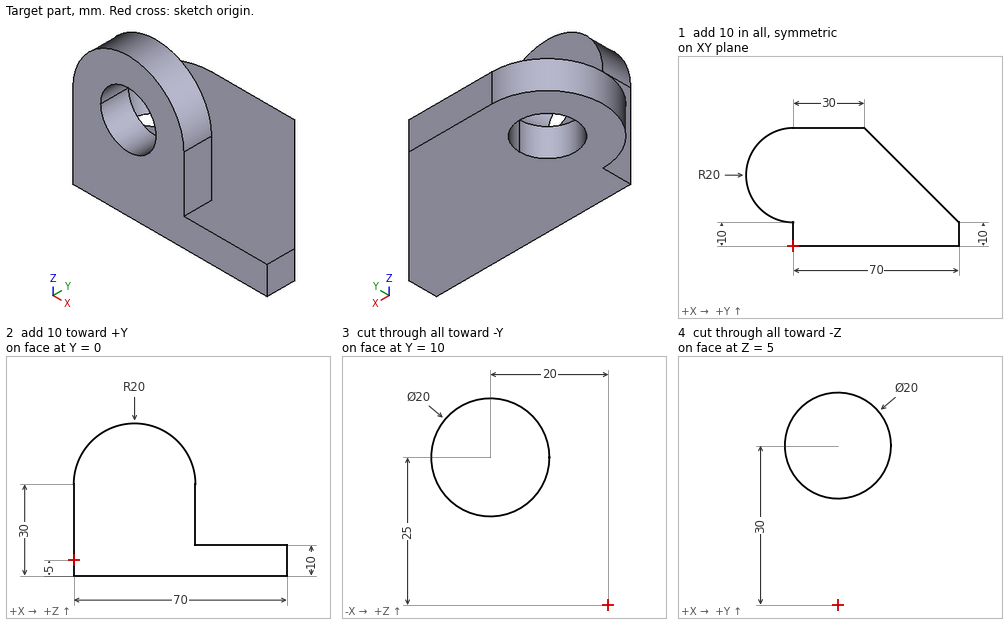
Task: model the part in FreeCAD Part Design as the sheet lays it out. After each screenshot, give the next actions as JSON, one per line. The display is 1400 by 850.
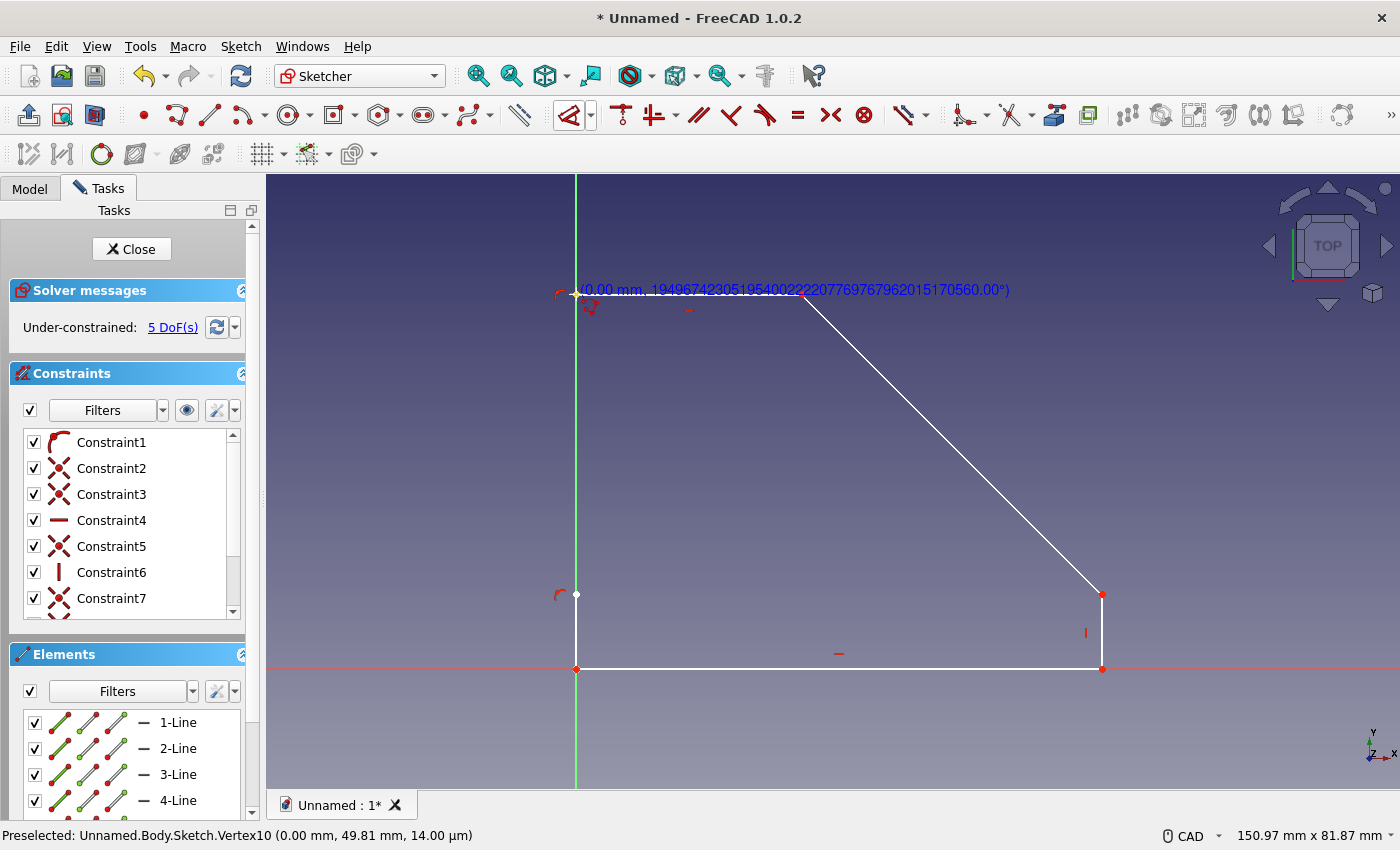
{"action": "key", "text": "g 3 a"}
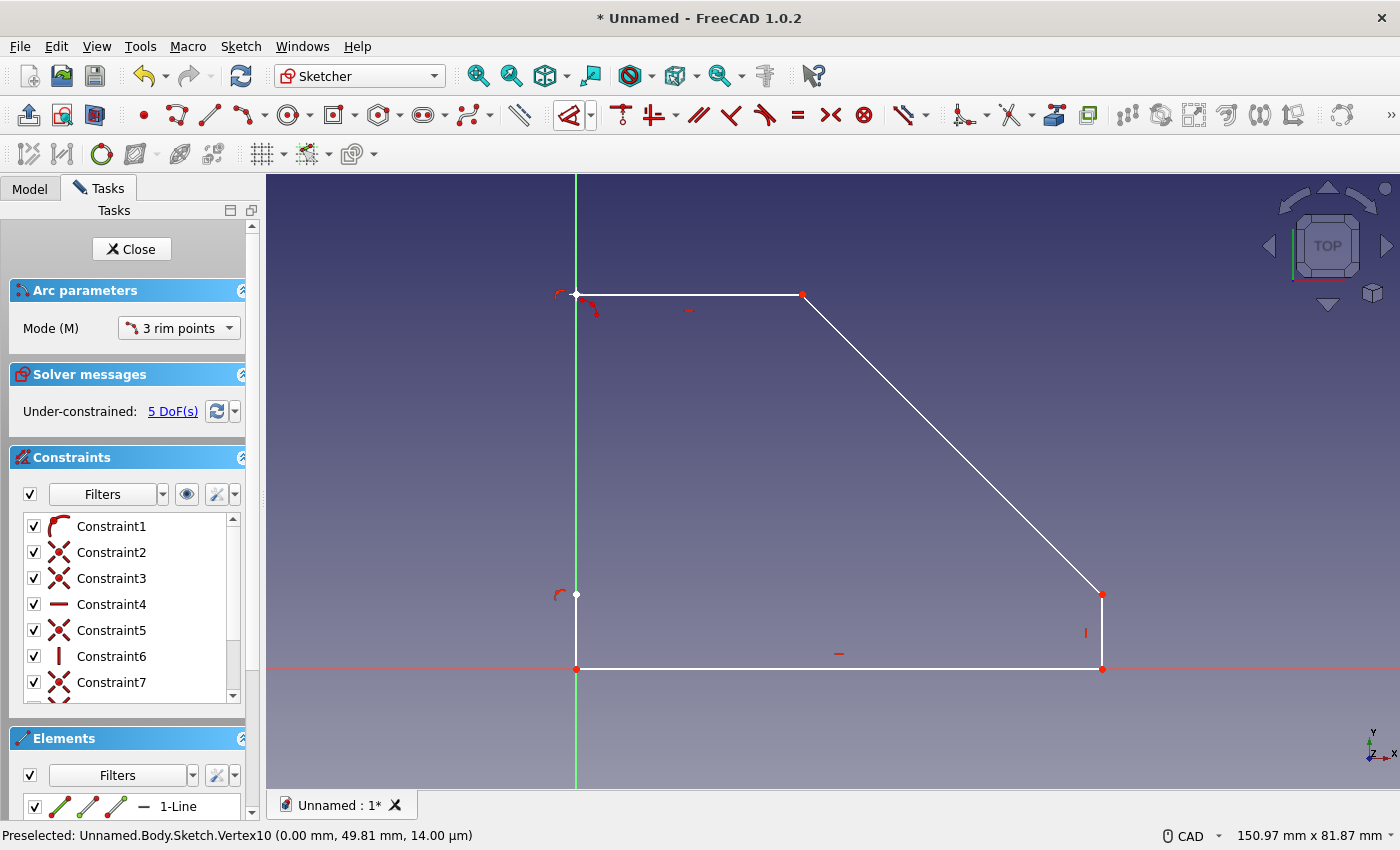
{"action": "left_click", "coordinate": [576, 295]}
{"action": "left_click", "coordinate": [576, 595]}
{"action": "left_click", "coordinate": [426, 444]}
{"action": "key", "text": "Escape"}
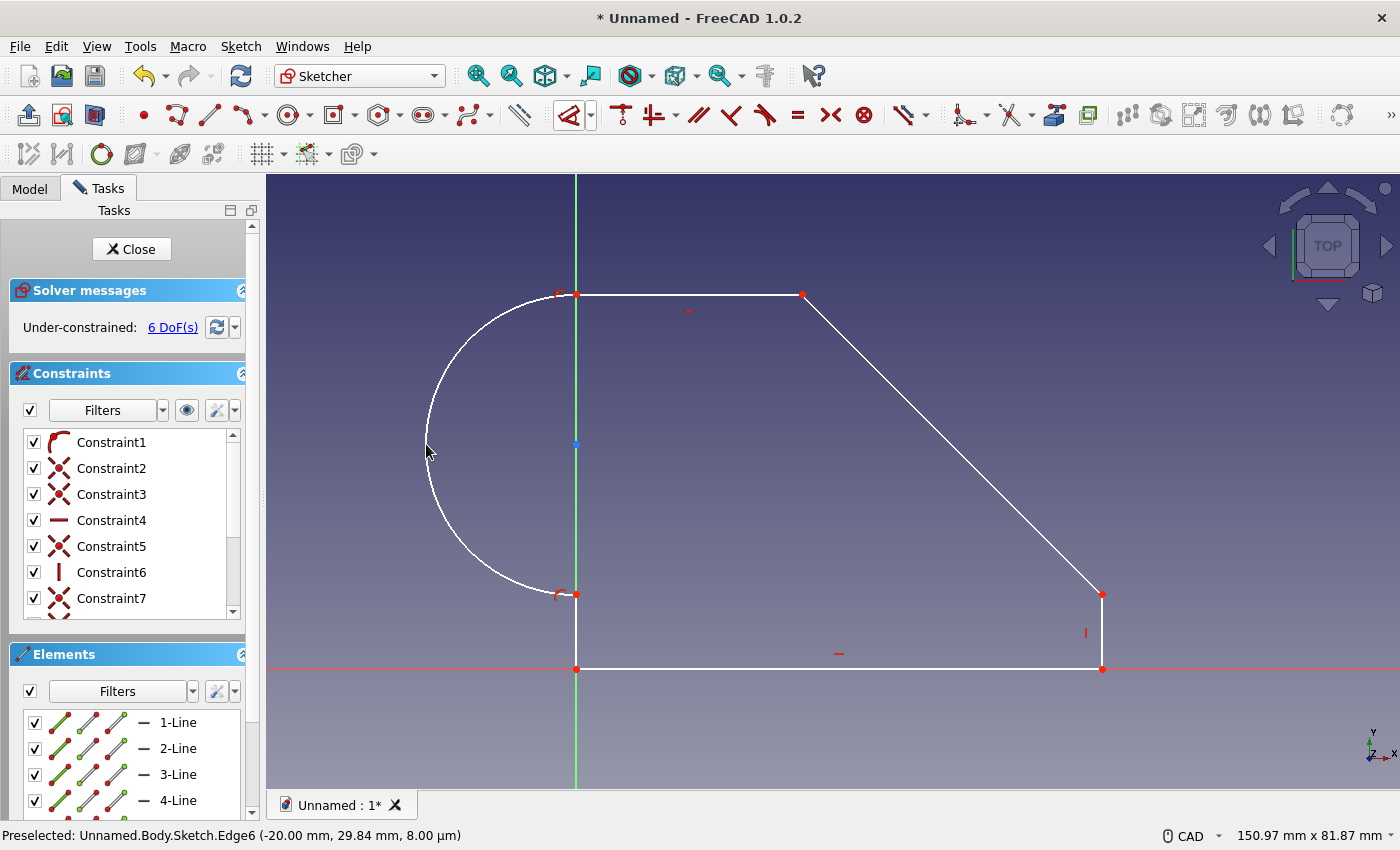
{"action": "left_click", "coordinate": [734, 295]}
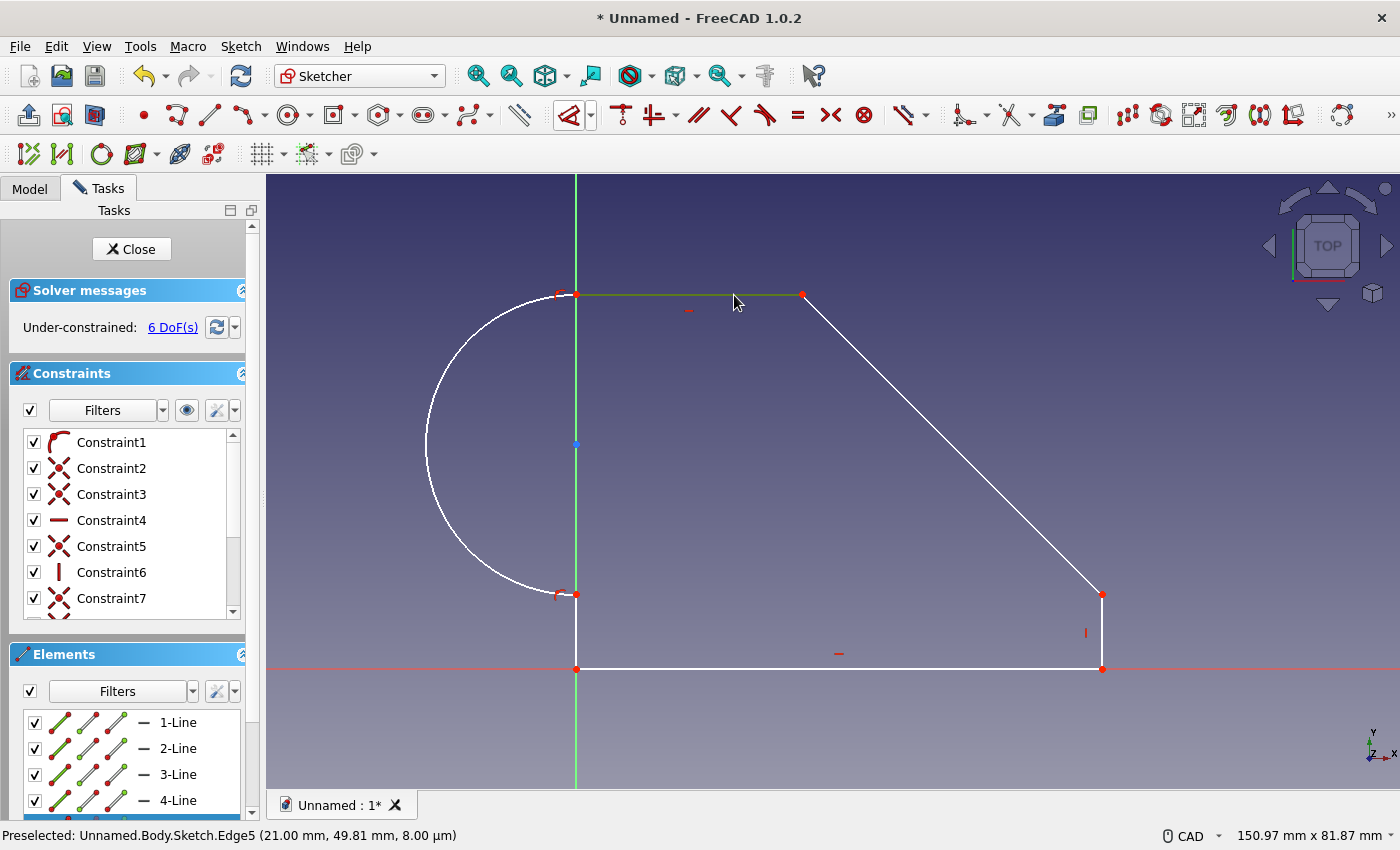
{"action": "left_click", "coordinate": [455, 357]}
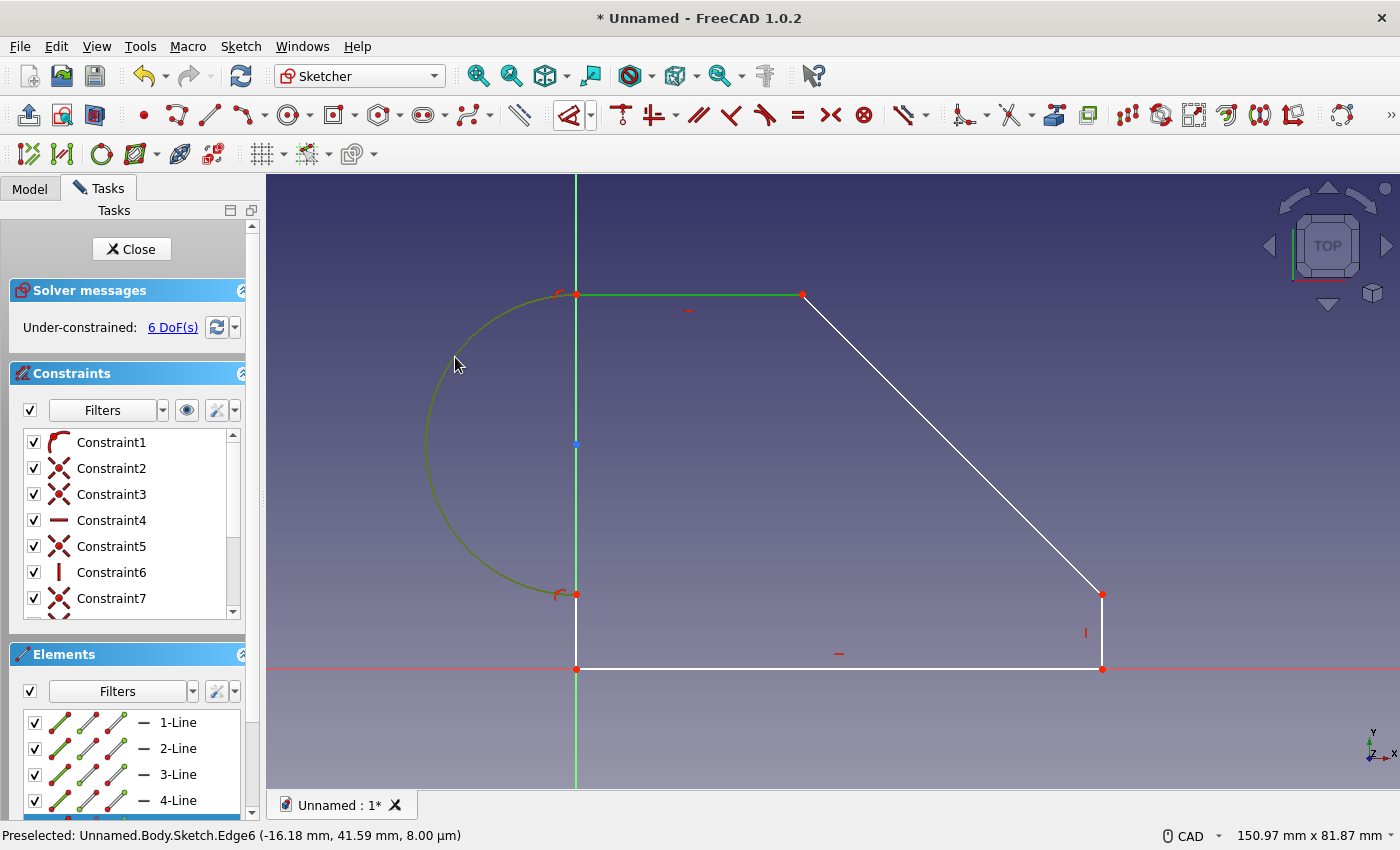
{"action": "left_click", "coordinate": [765, 116]}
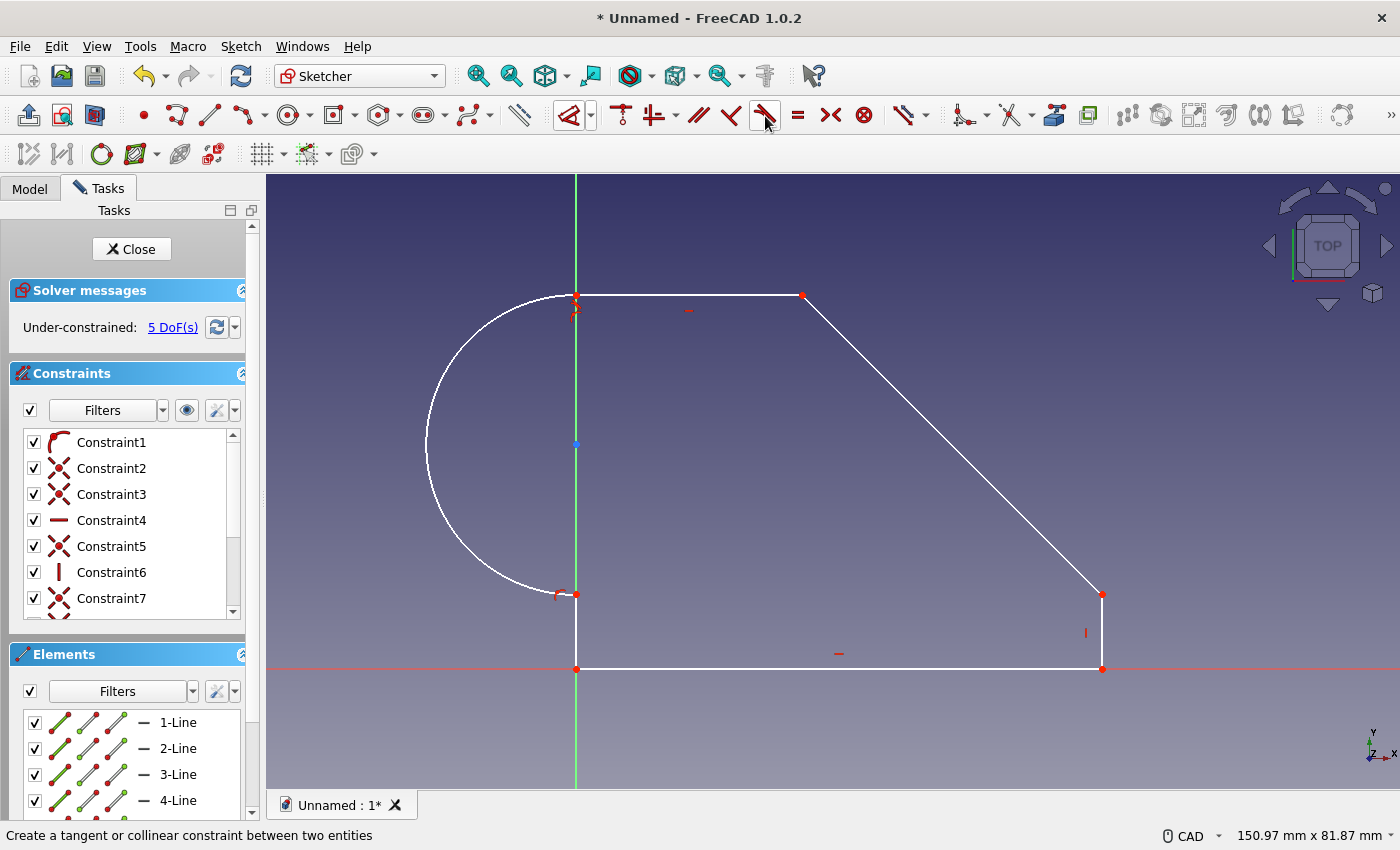
{"action": "left_click", "coordinate": [455, 357]}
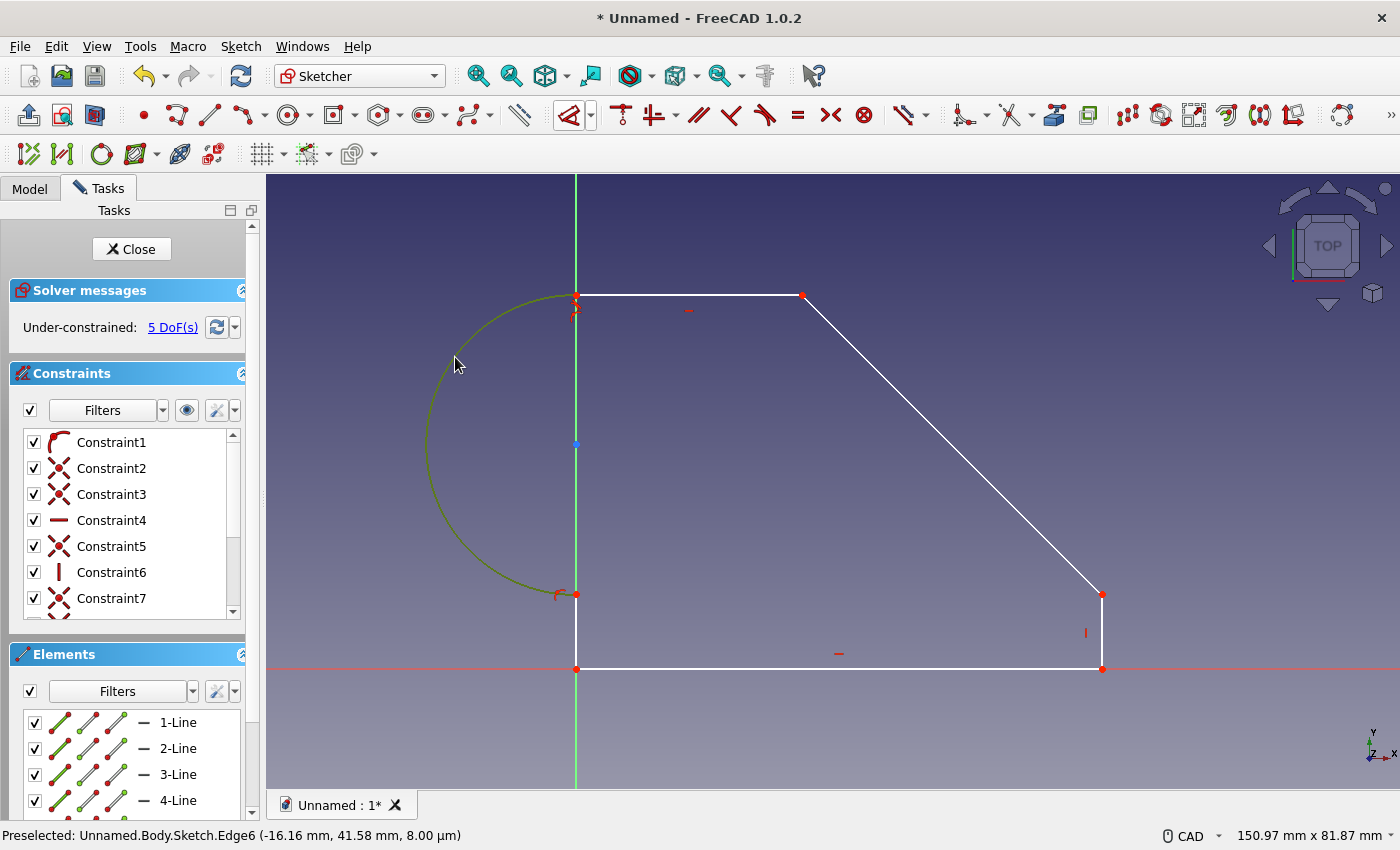
{"action": "key", "text": "k r"}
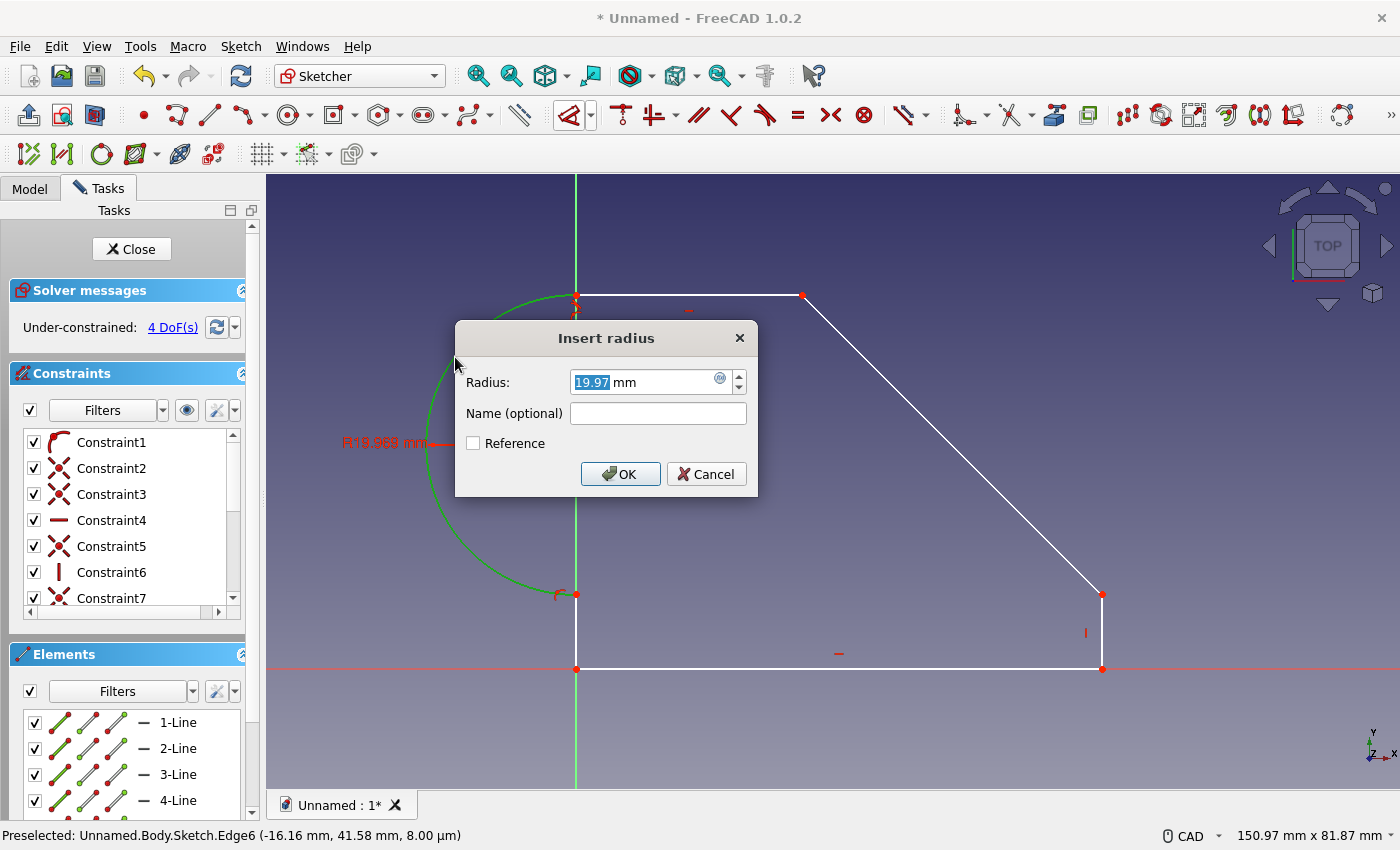
{"action": "type", "text": "20"}
{"action": "key", "text": "Return"}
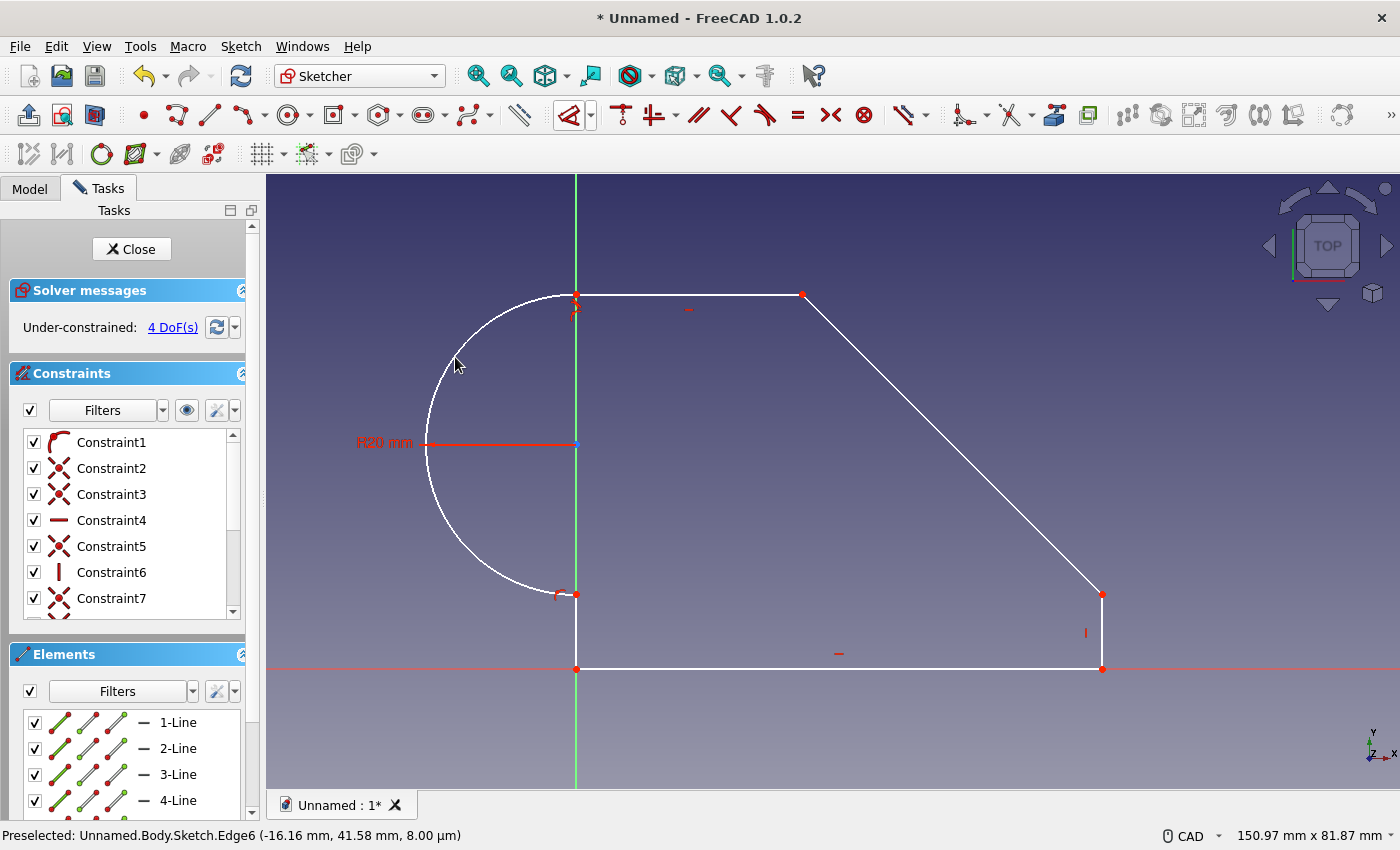
{"action": "left_click", "coordinate": [576, 617]}